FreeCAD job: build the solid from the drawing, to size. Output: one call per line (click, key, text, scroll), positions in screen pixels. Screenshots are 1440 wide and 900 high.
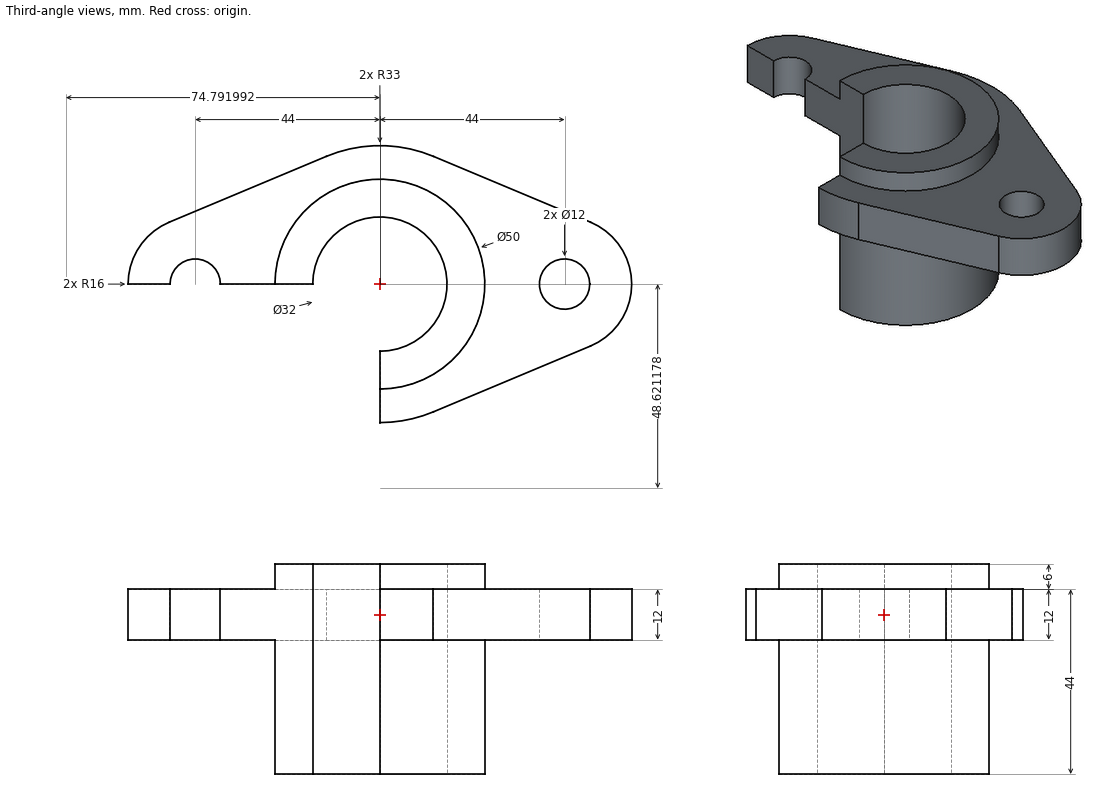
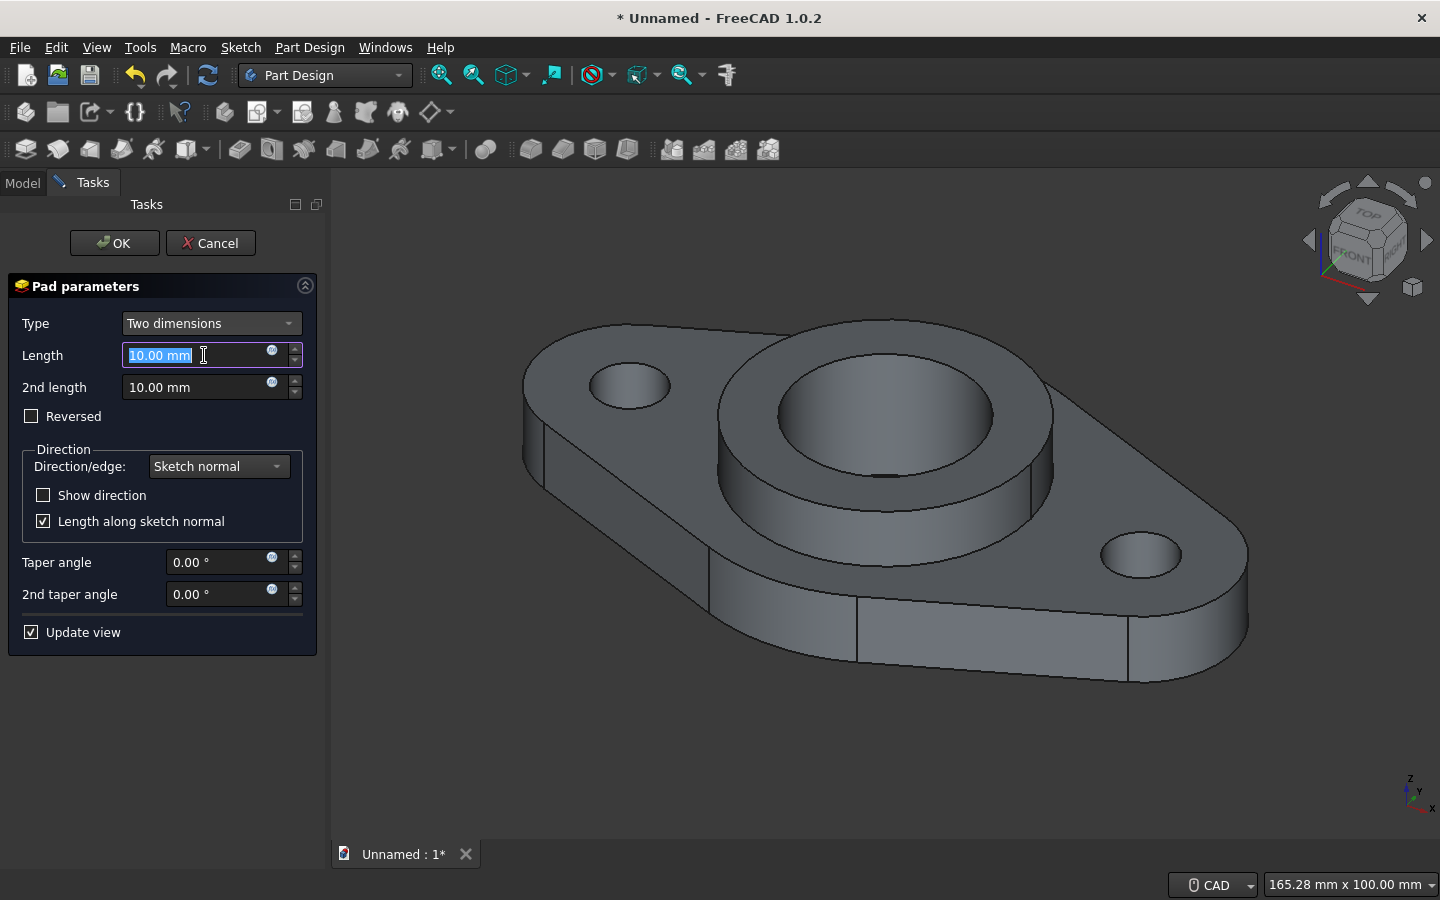
text(6)
key(Tab)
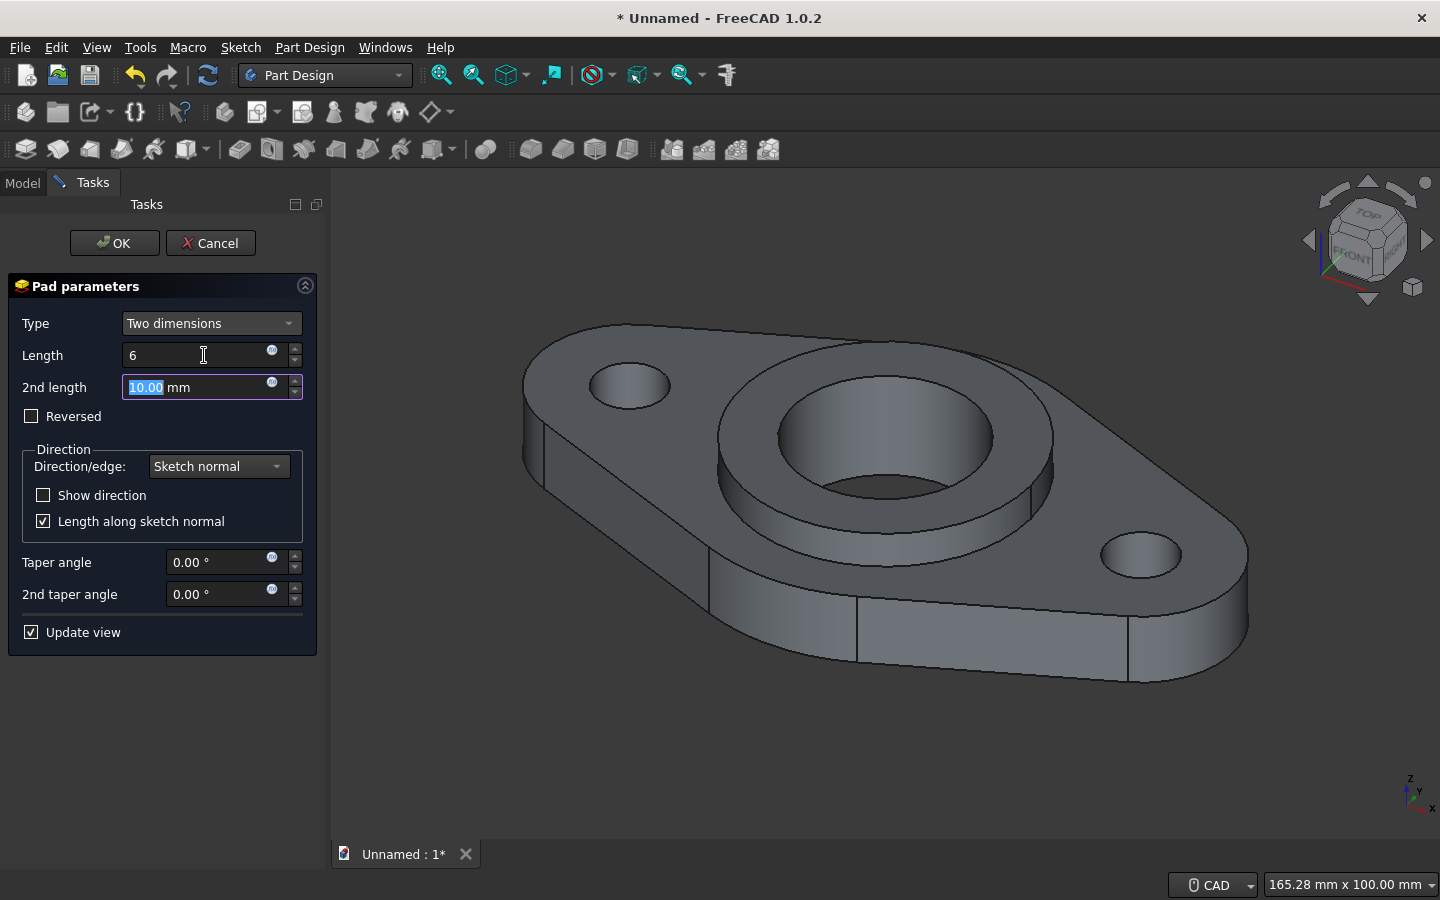
text(44)
key(Tab)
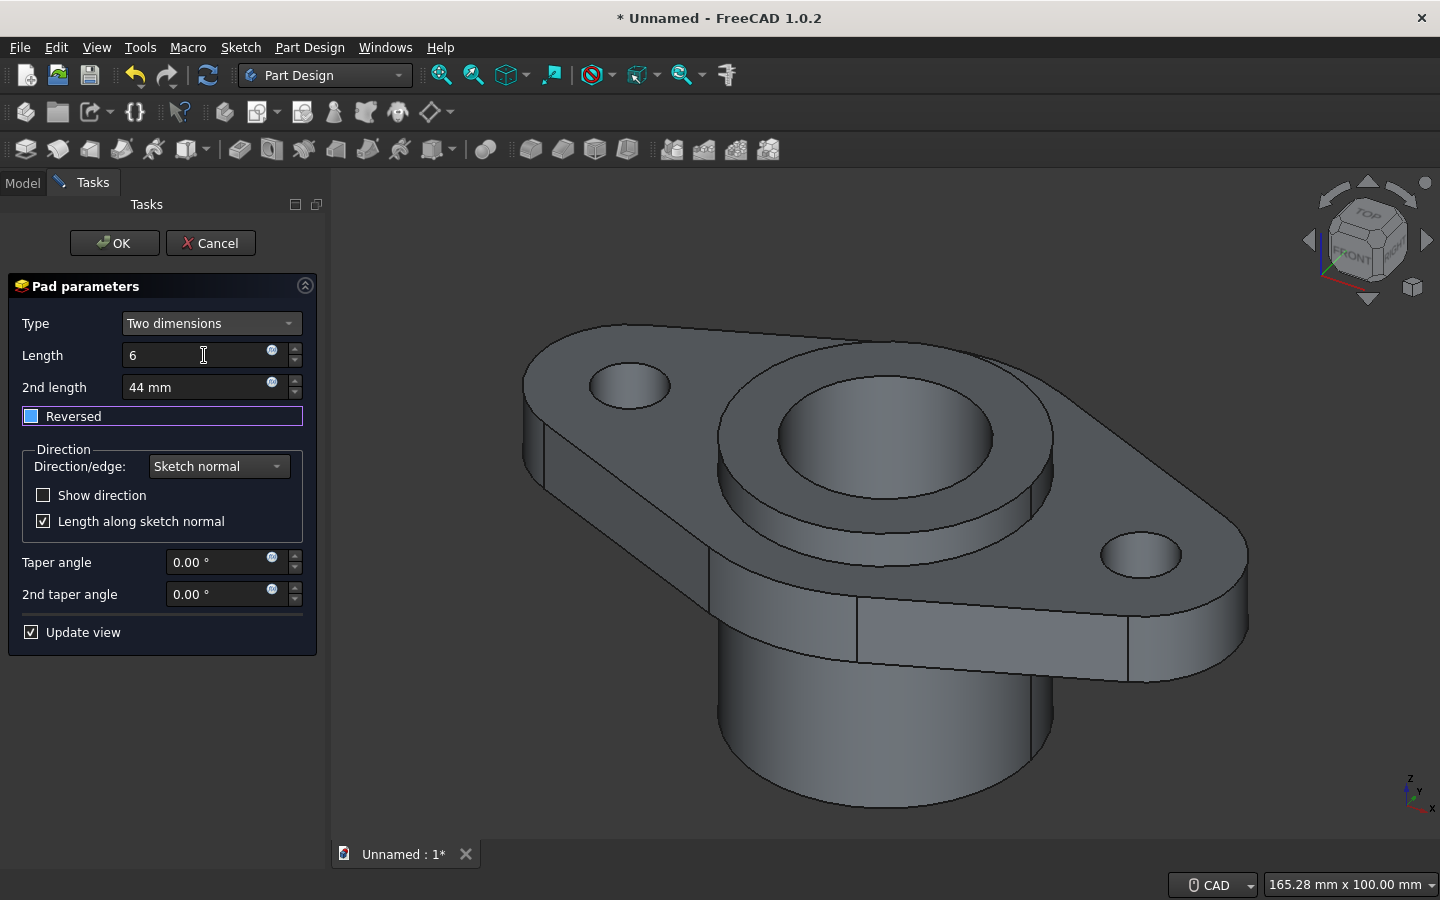
click(115, 243)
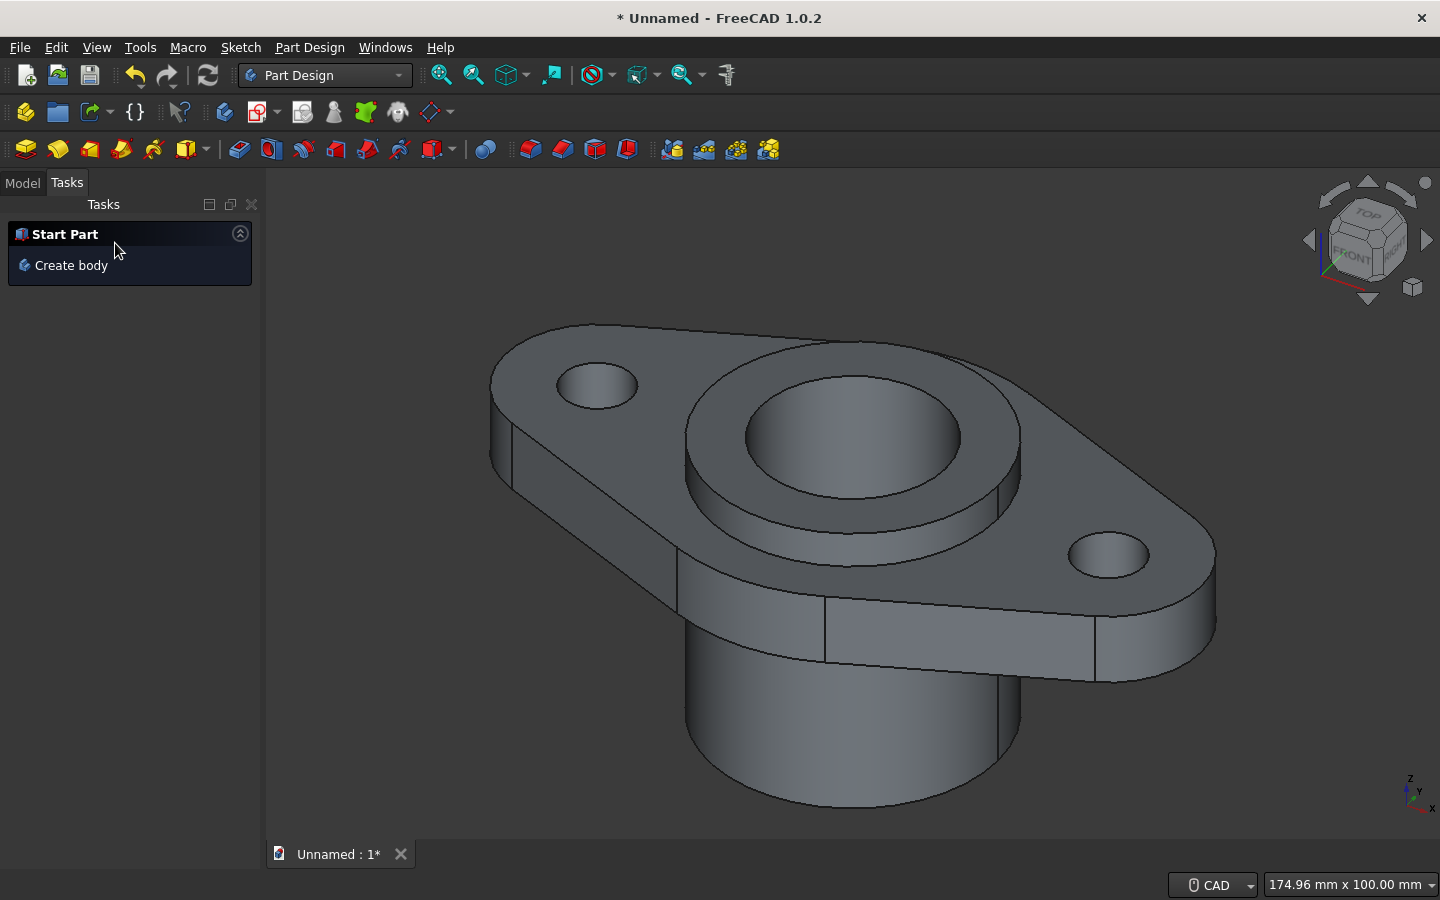
click(442, 76)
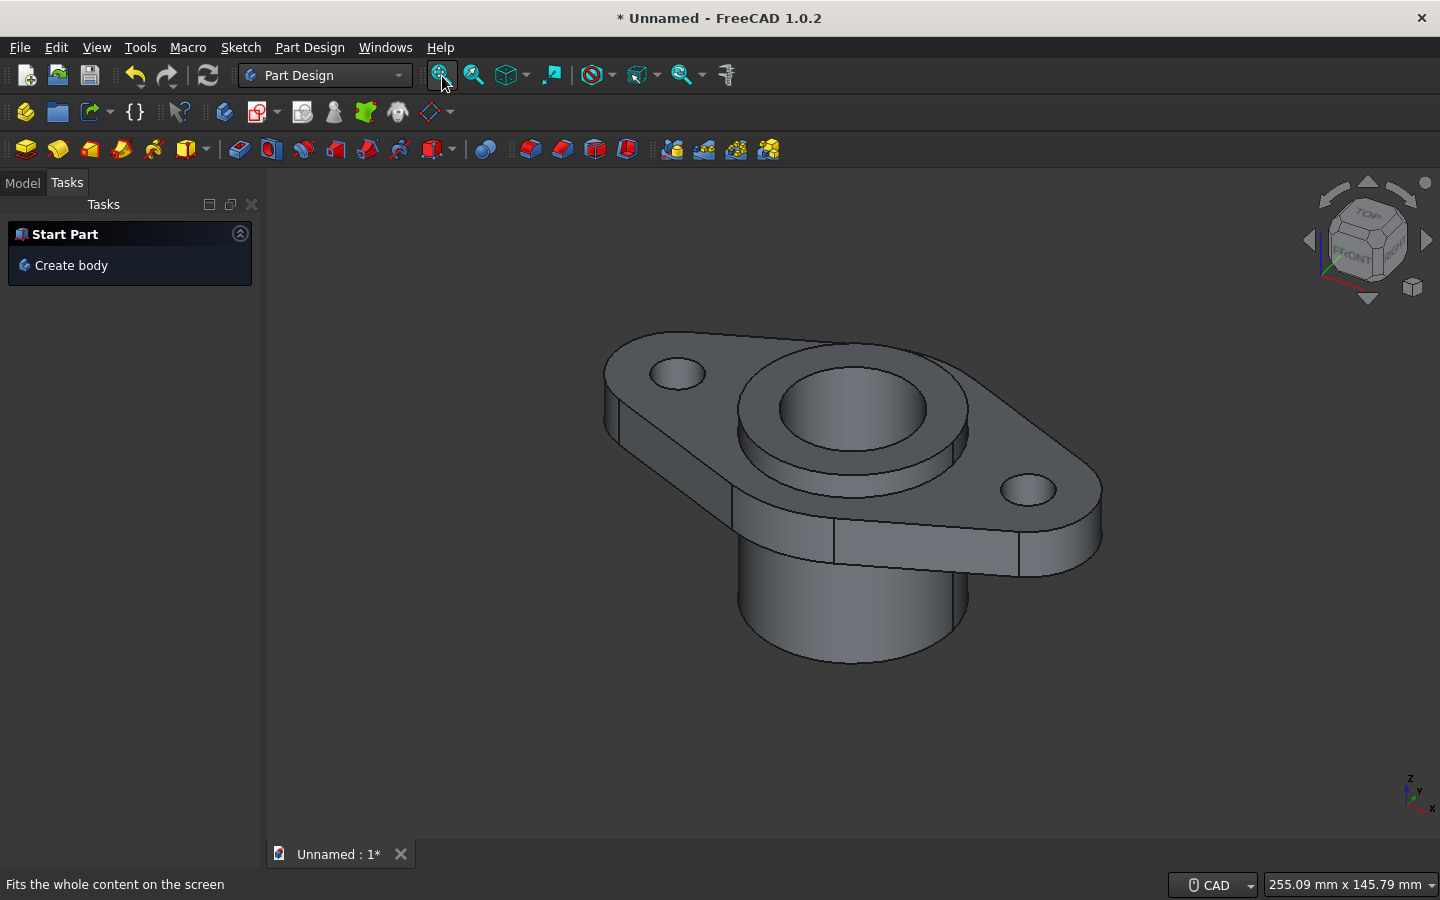
key(5)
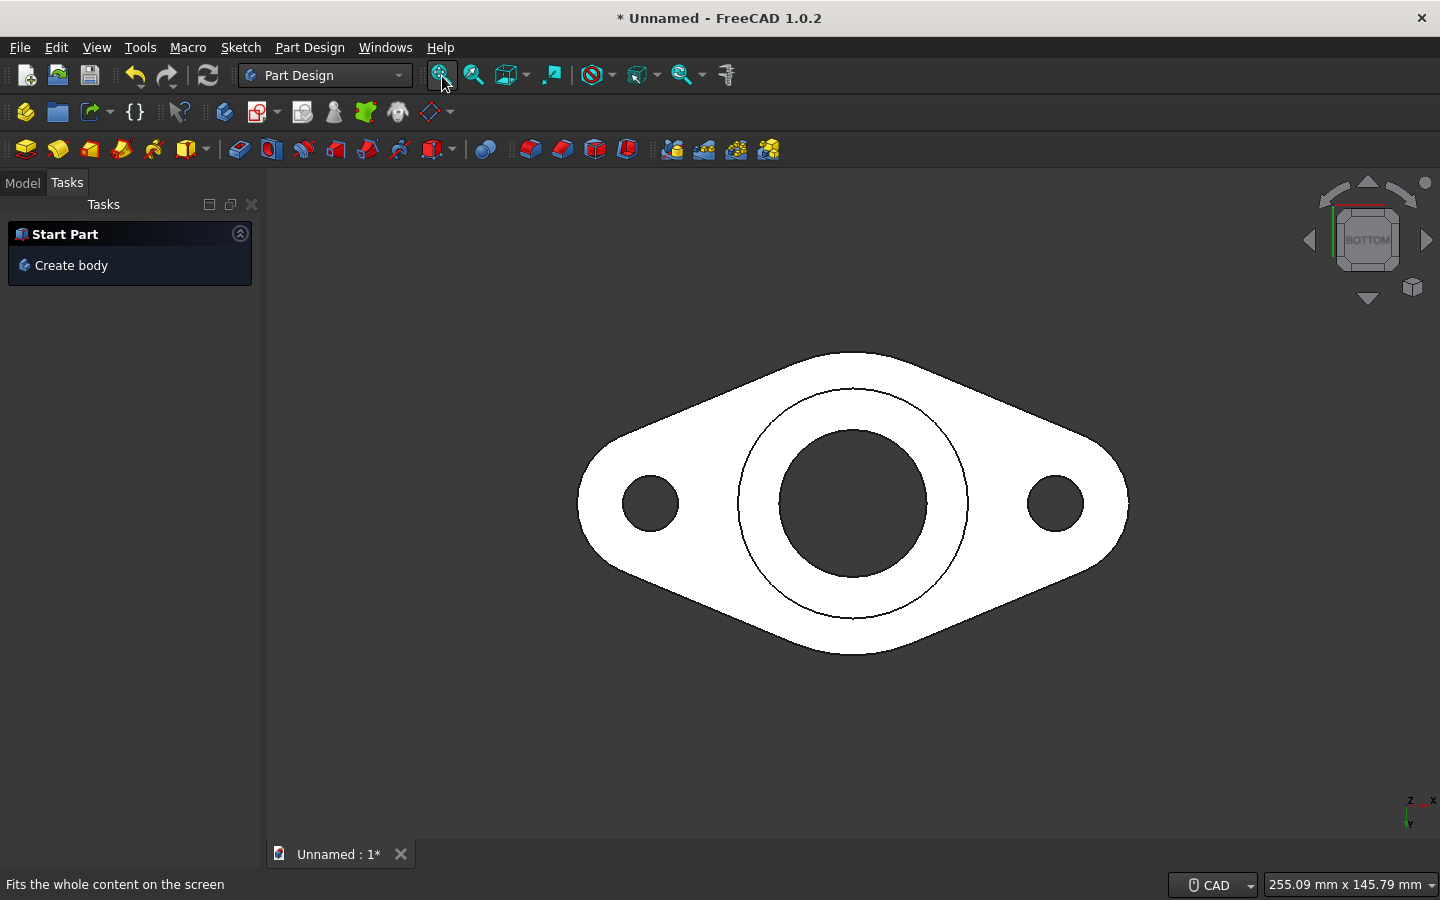
click(787, 568)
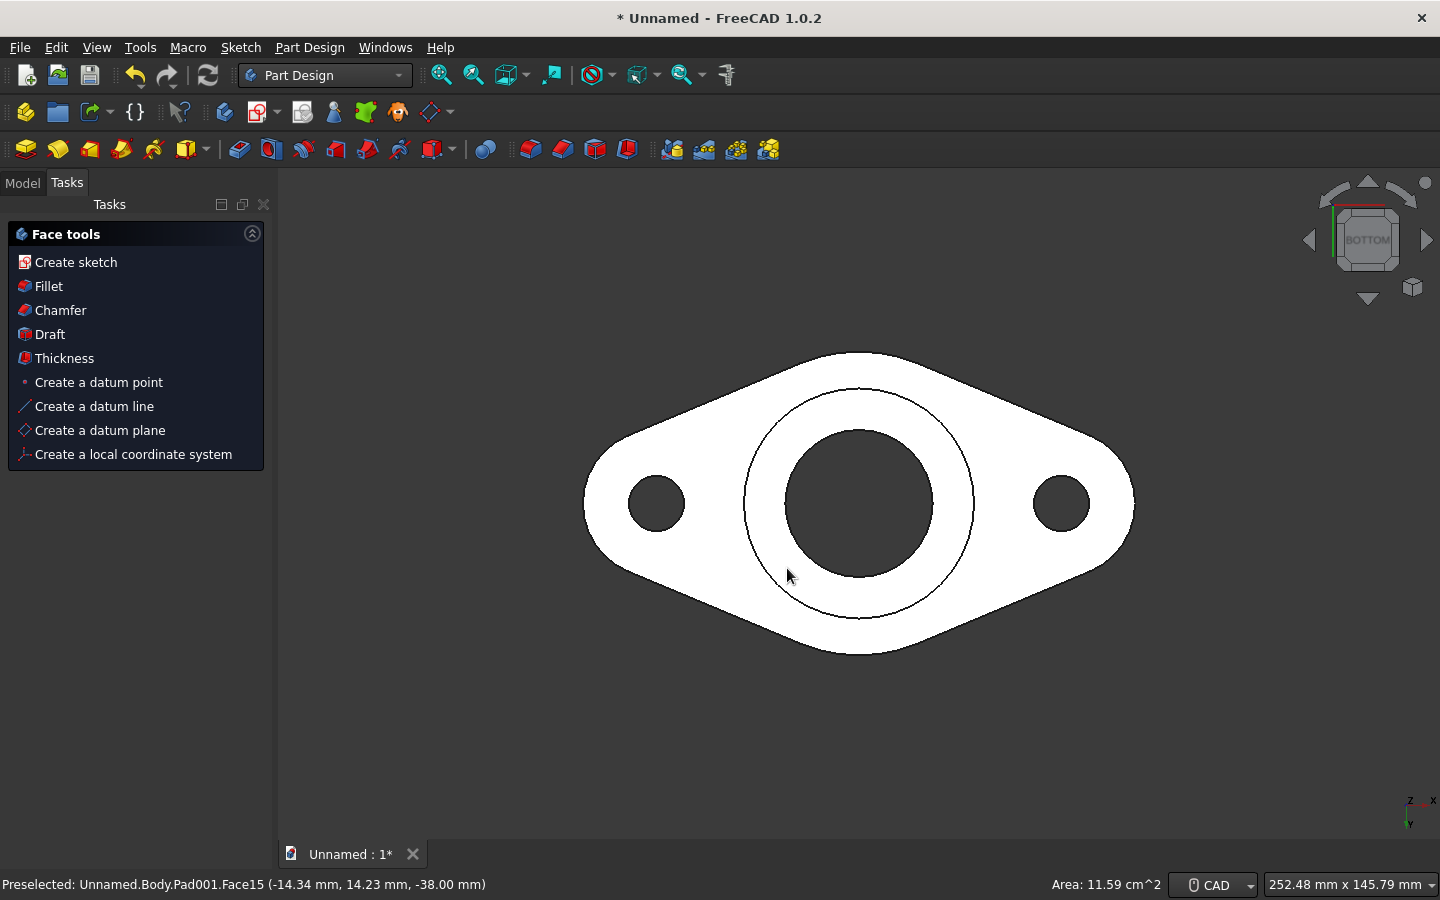
click(258, 112)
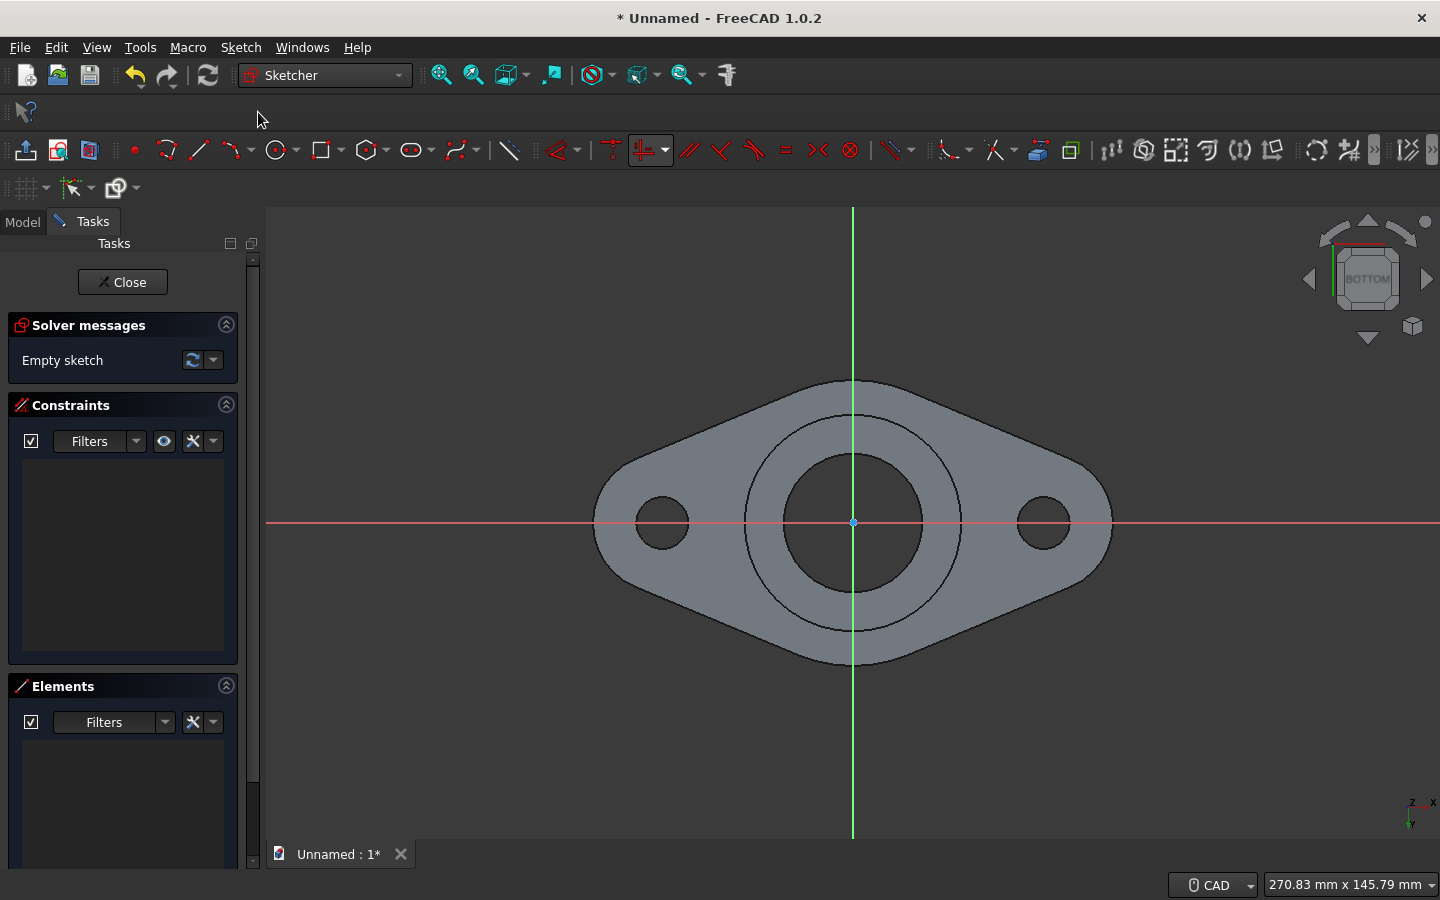
scroll(577, 289, up, 3)